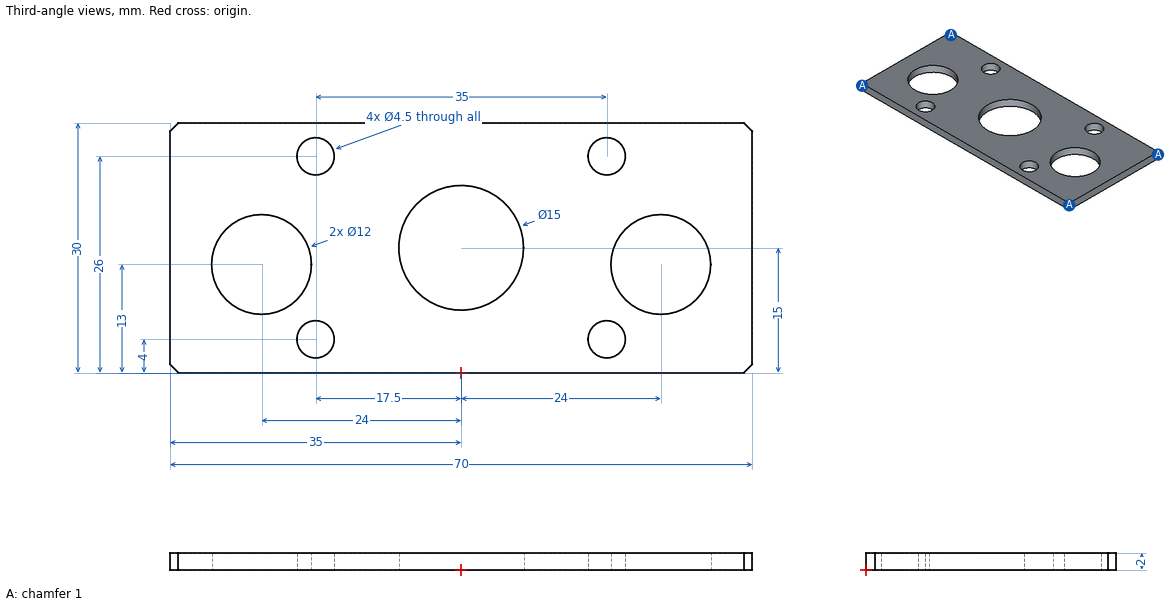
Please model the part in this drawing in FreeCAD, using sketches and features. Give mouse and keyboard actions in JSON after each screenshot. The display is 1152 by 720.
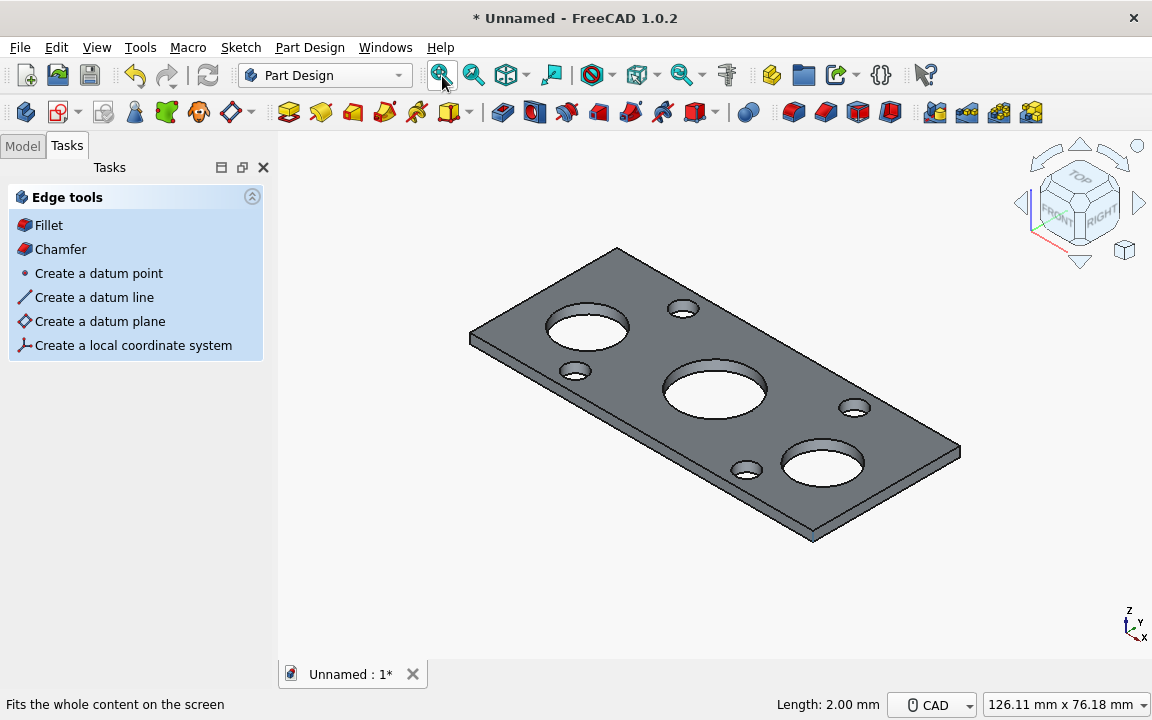
{"action": "scroll", "coordinate": [470, 337], "scroll_direction": "up", "scroll_amount": 6}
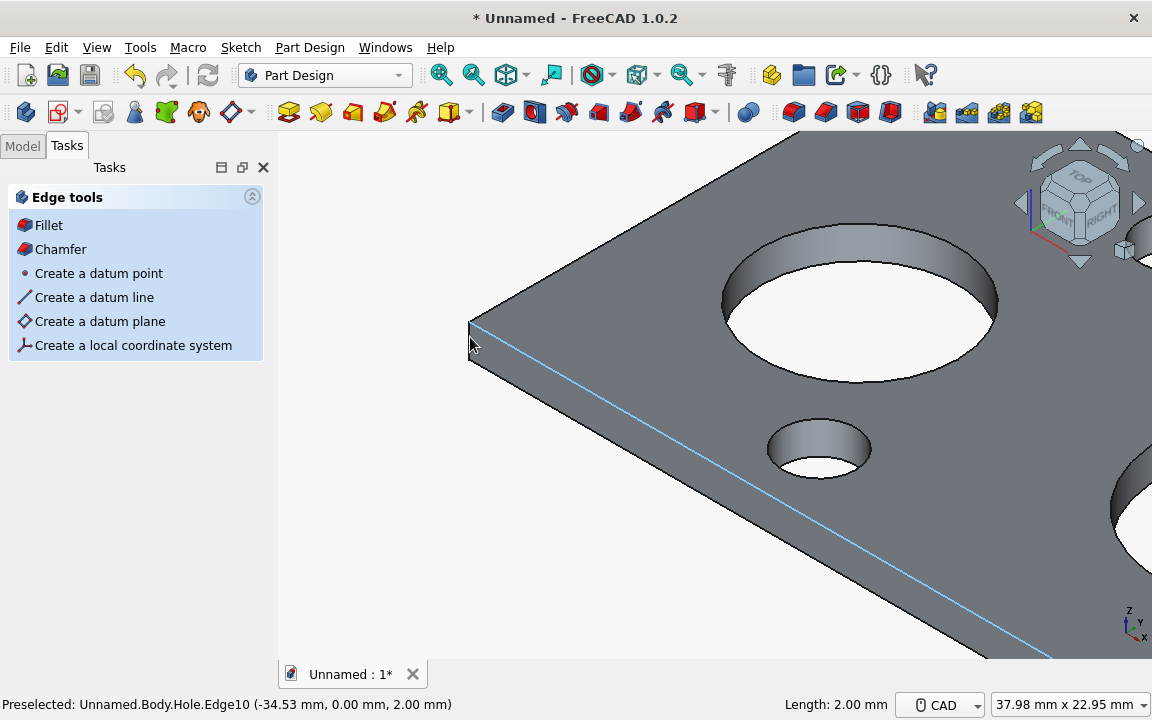
{"action": "left_click", "coordinate": [442, 76]}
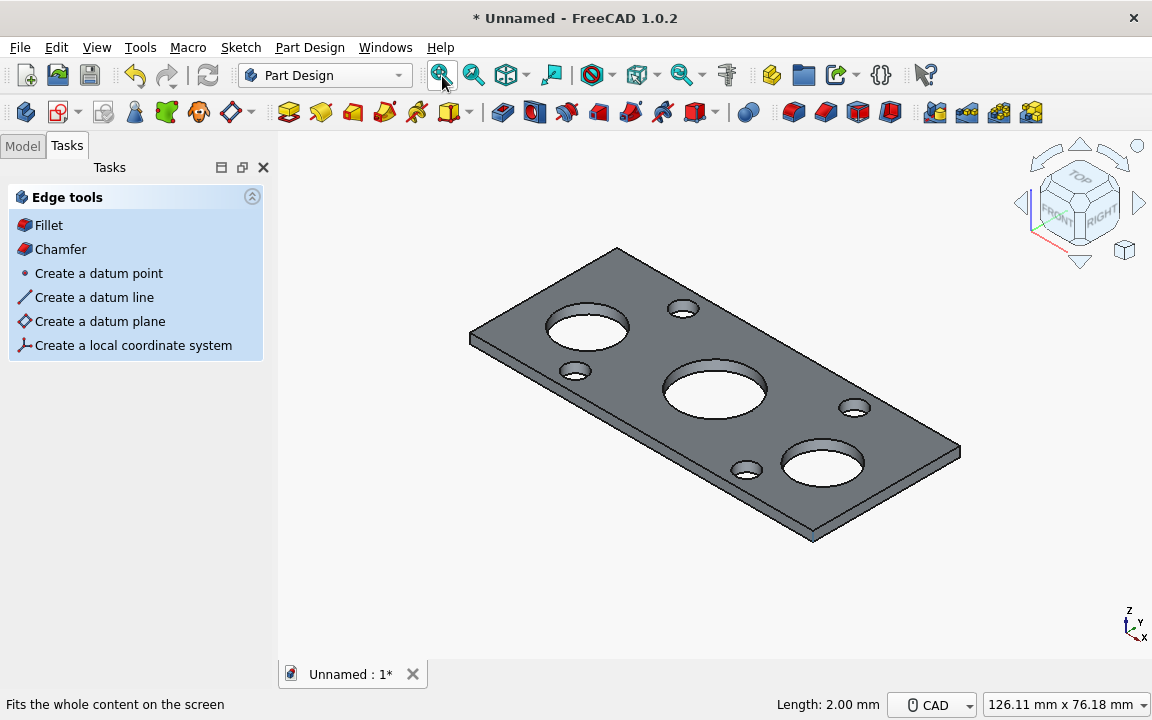
{"action": "key", "text": "2"}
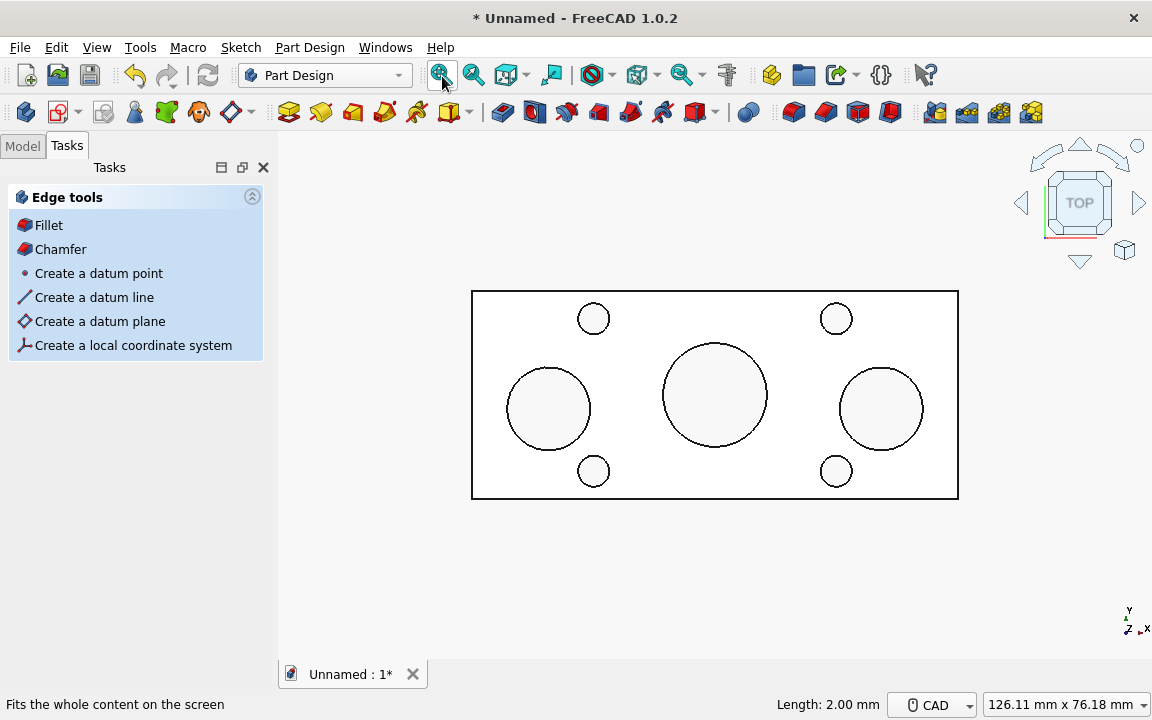
{"action": "scroll", "coordinate": [472, 498], "scroll_direction": "up", "scroll_amount": 6}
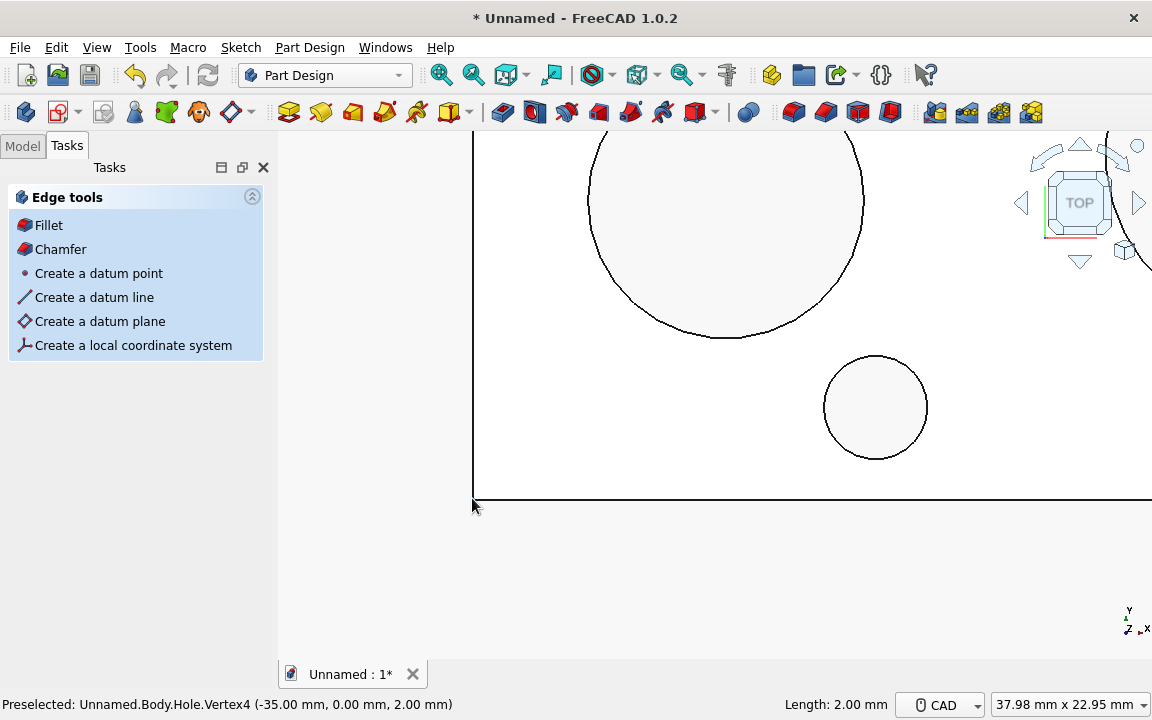
{"action": "left_click", "coordinate": [442, 76]}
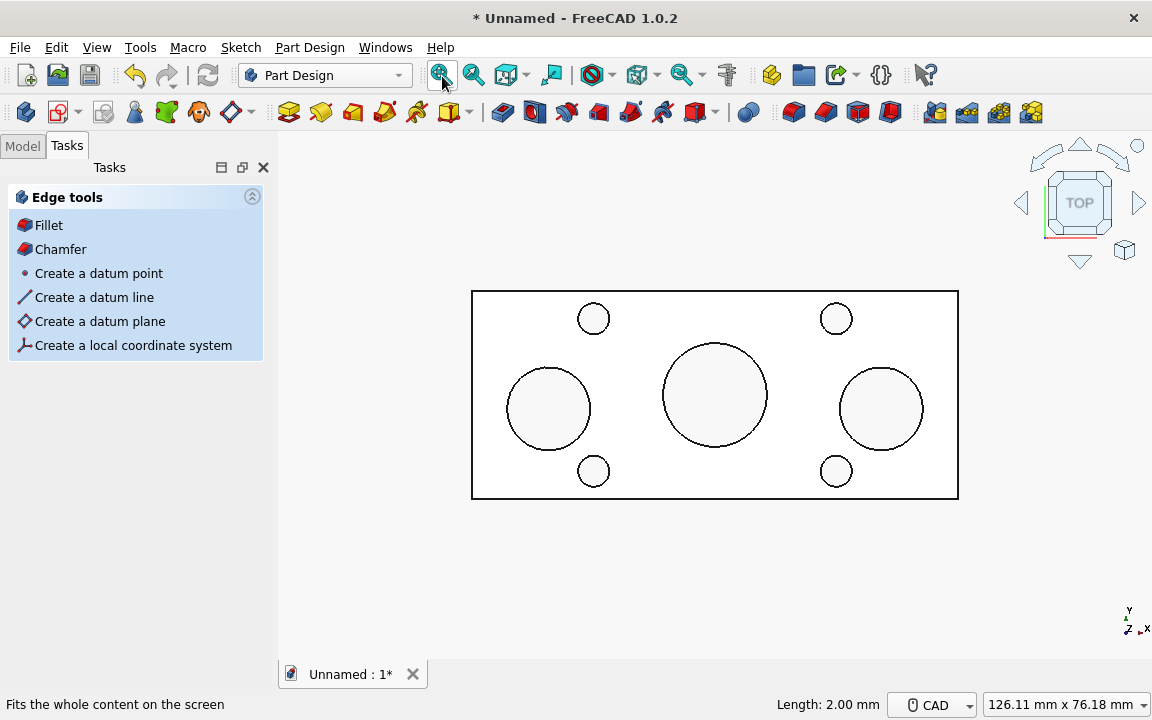
{"action": "key", "text": "1"}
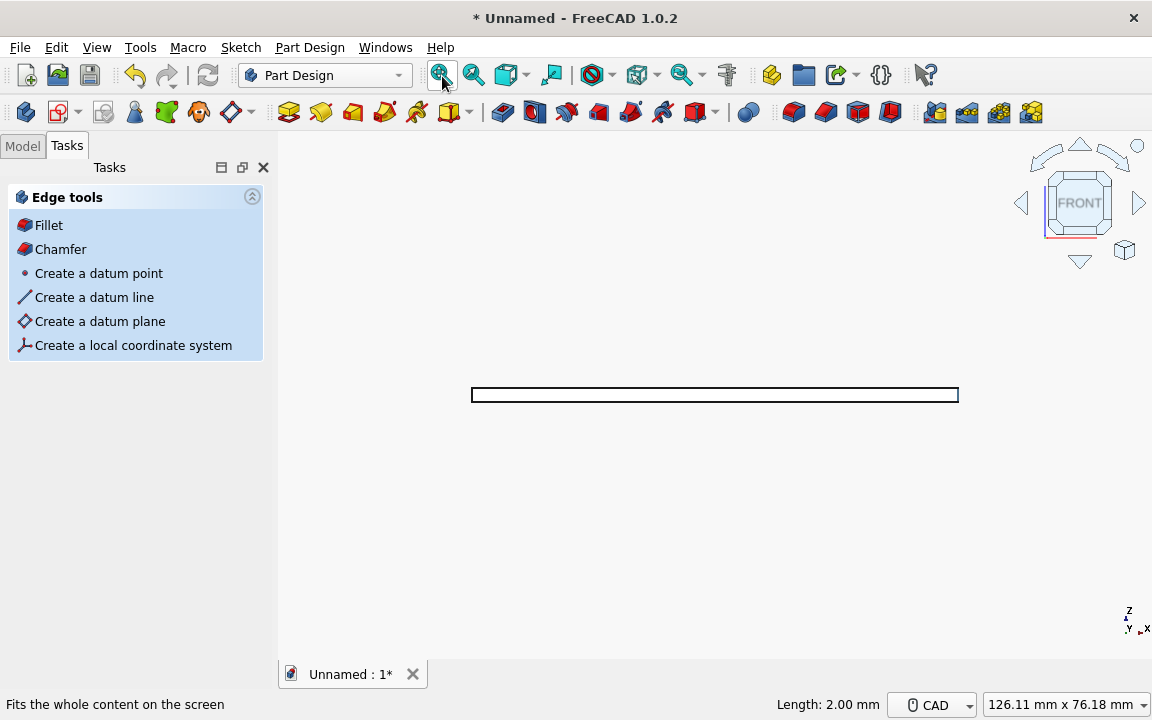
{"action": "left_click", "coordinate": [472, 394], "text": "ctrl"}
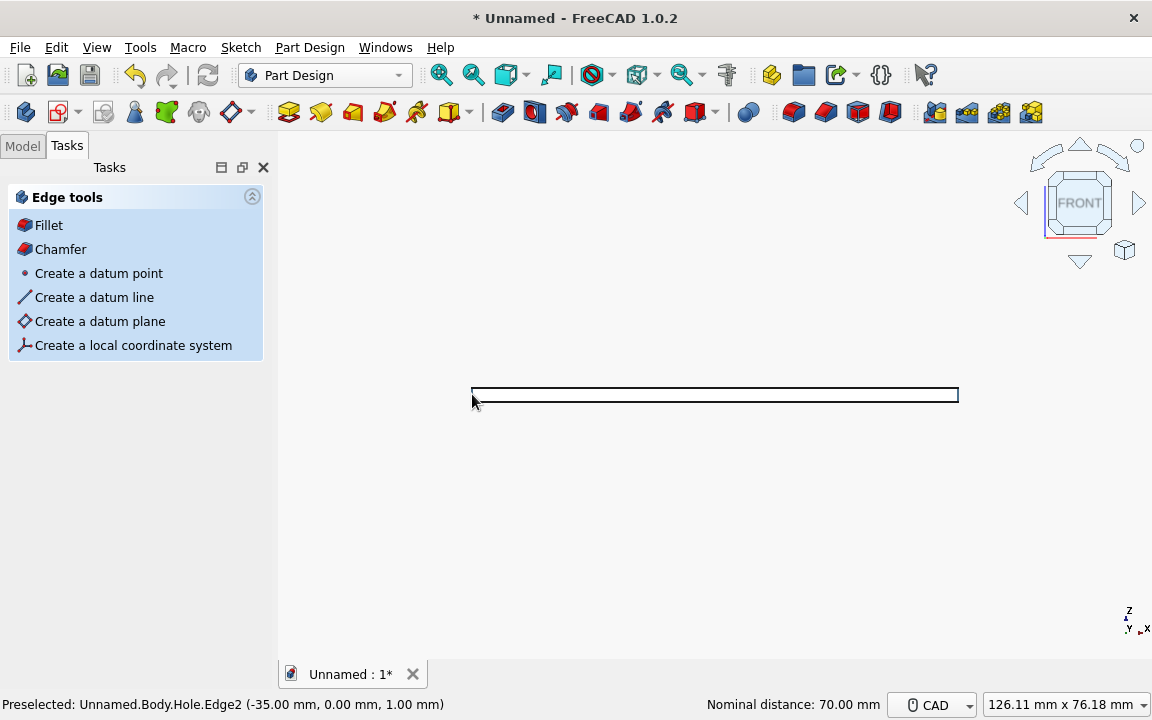
{"action": "scroll", "coordinate": [472, 394], "scroll_direction": "up", "scroll_amount": 6}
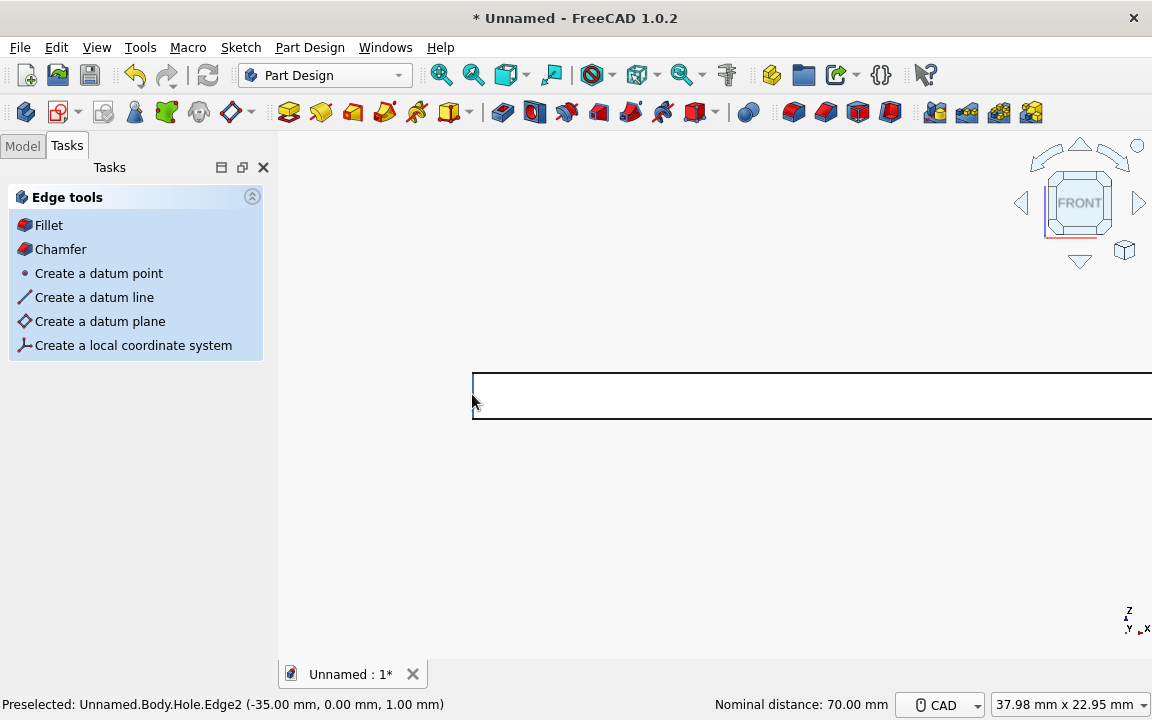
{"action": "left_click", "coordinate": [442, 76]}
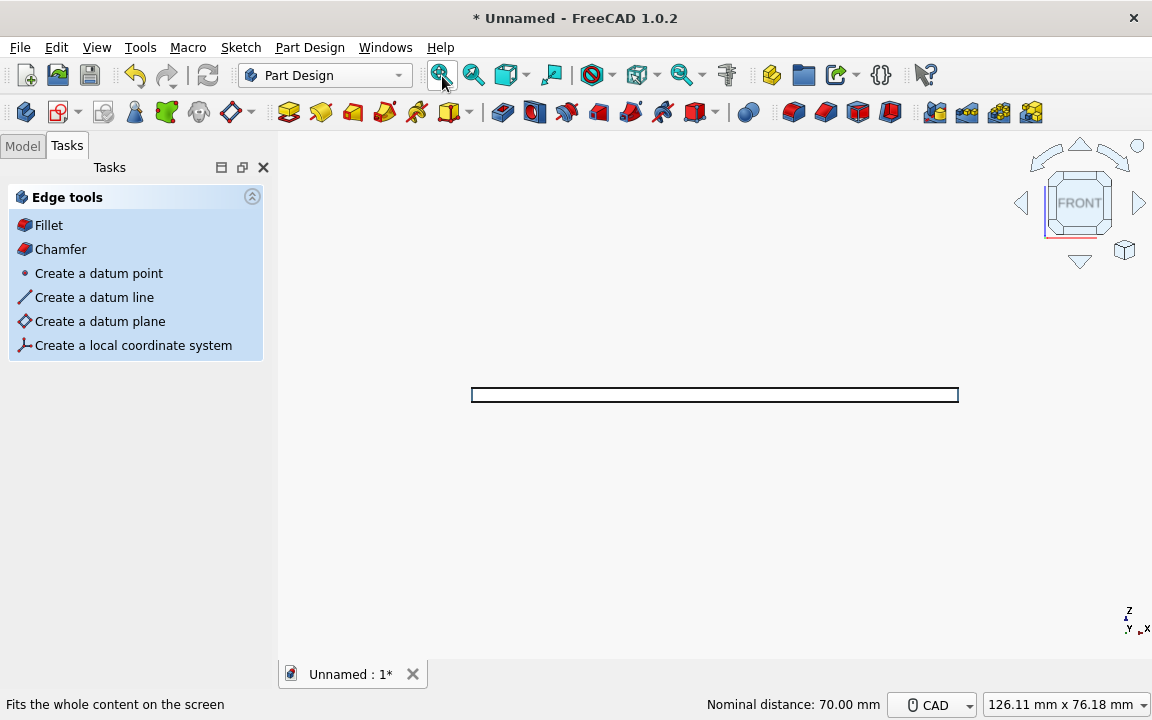
{"action": "key", "text": "3"}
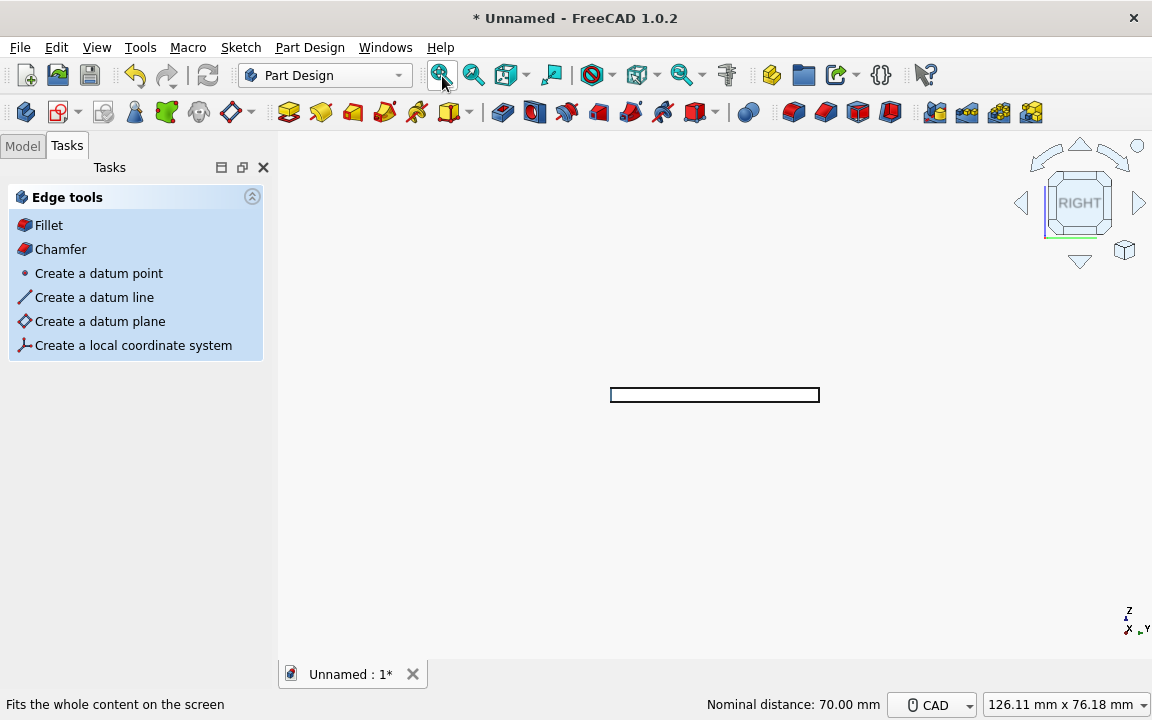
{"action": "left_click", "coordinate": [442, 76]}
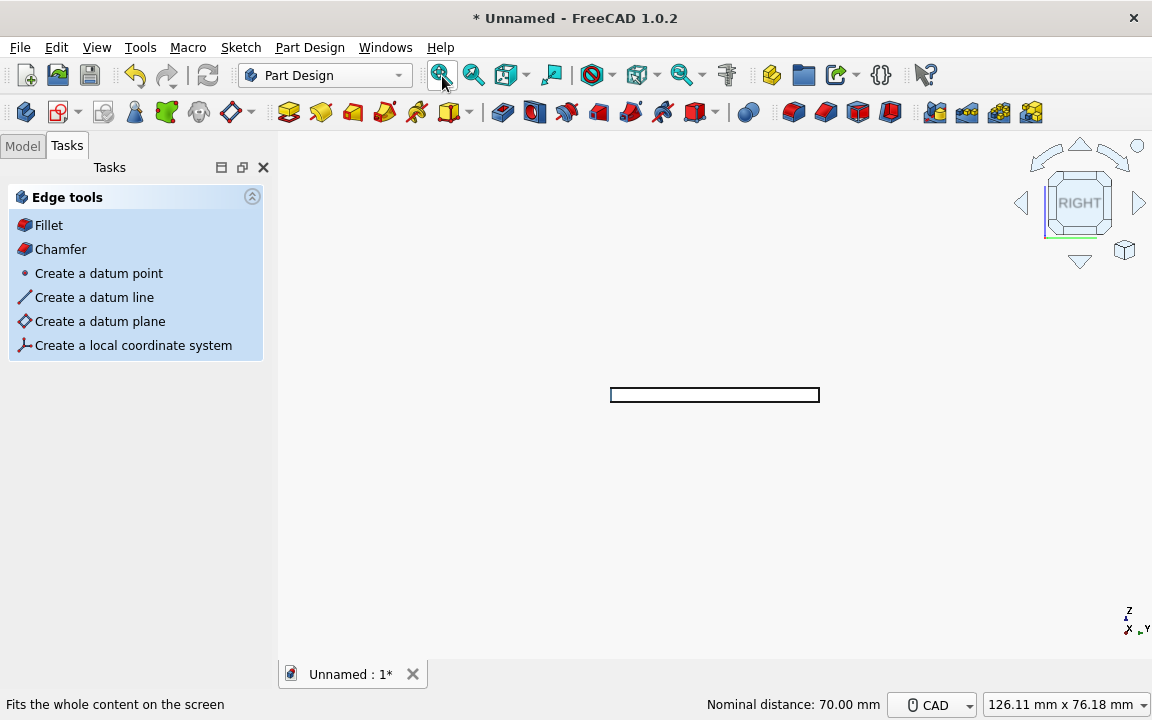
{"action": "left_click", "coordinate": [819, 394], "text": "ctrl"}